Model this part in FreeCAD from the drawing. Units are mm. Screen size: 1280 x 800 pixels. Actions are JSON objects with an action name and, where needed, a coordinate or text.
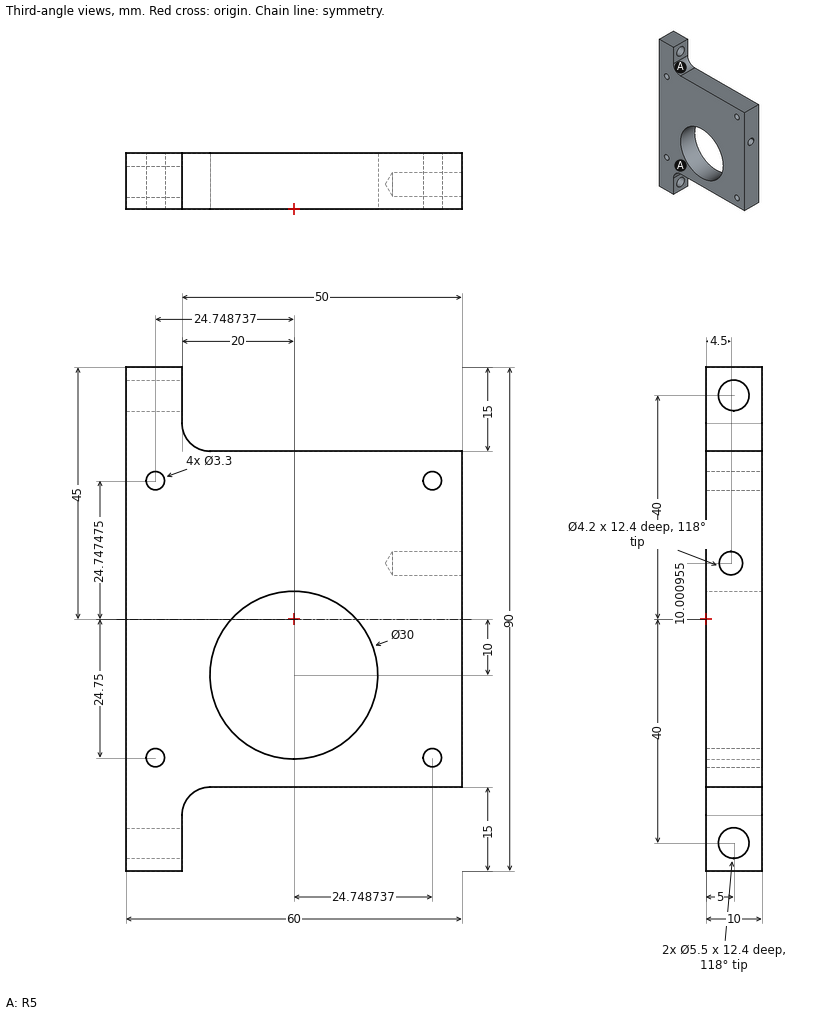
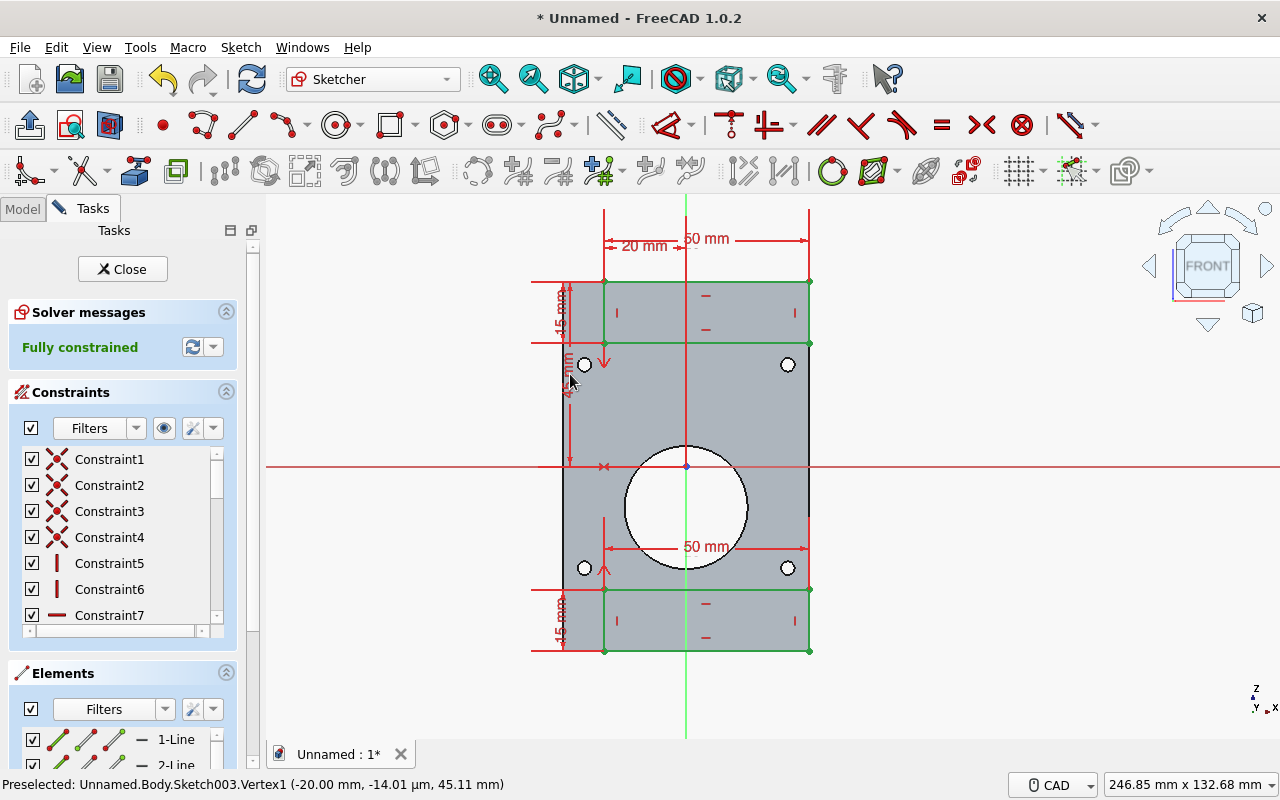
{"action": "left_click", "coordinate": [123, 269]}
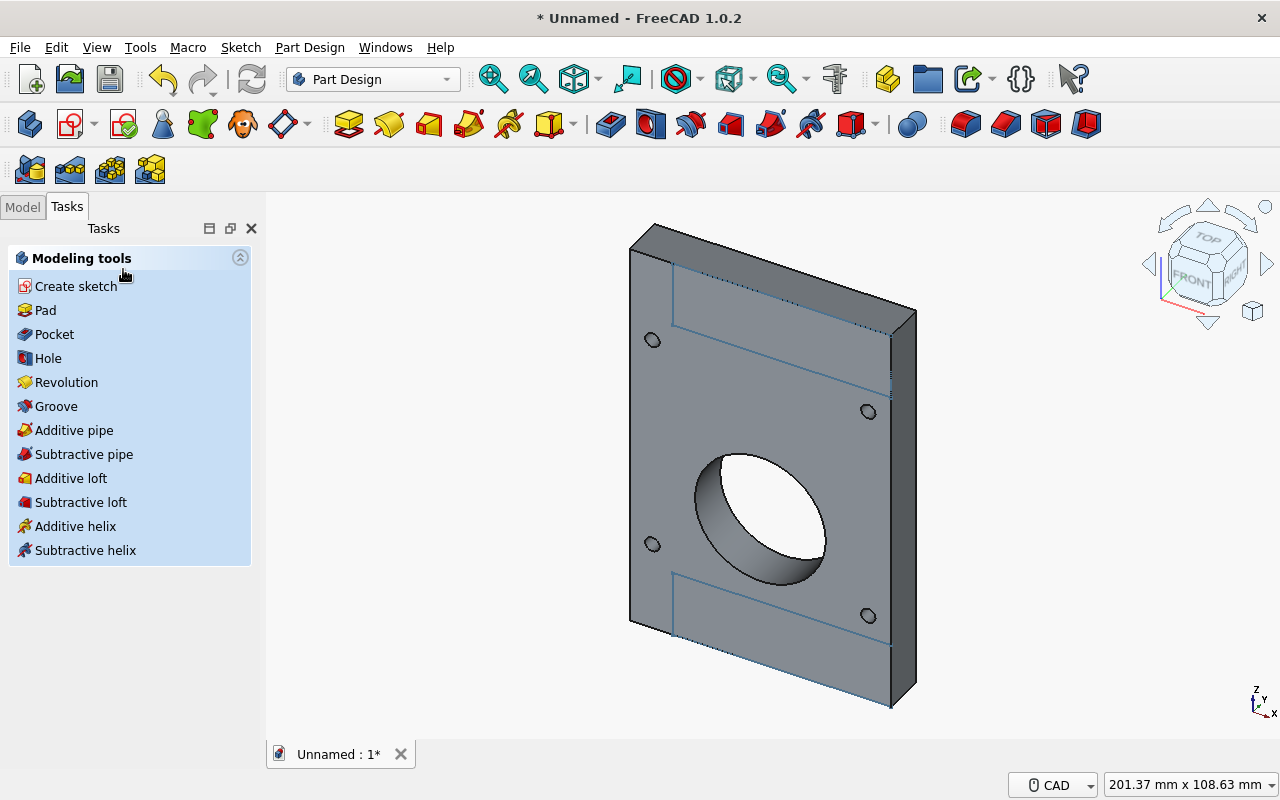
{"action": "left_click", "coordinate": [612, 124]}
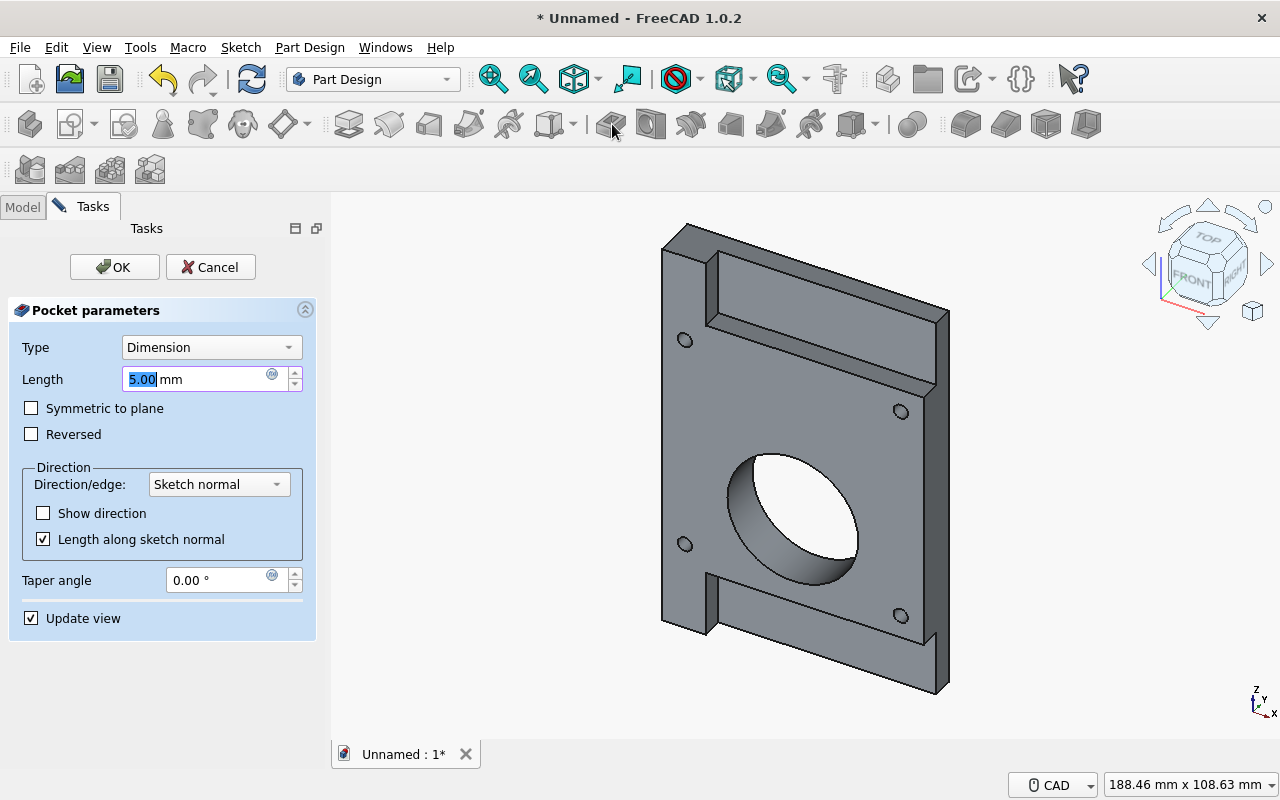
{"action": "left_click", "coordinate": [212, 348]}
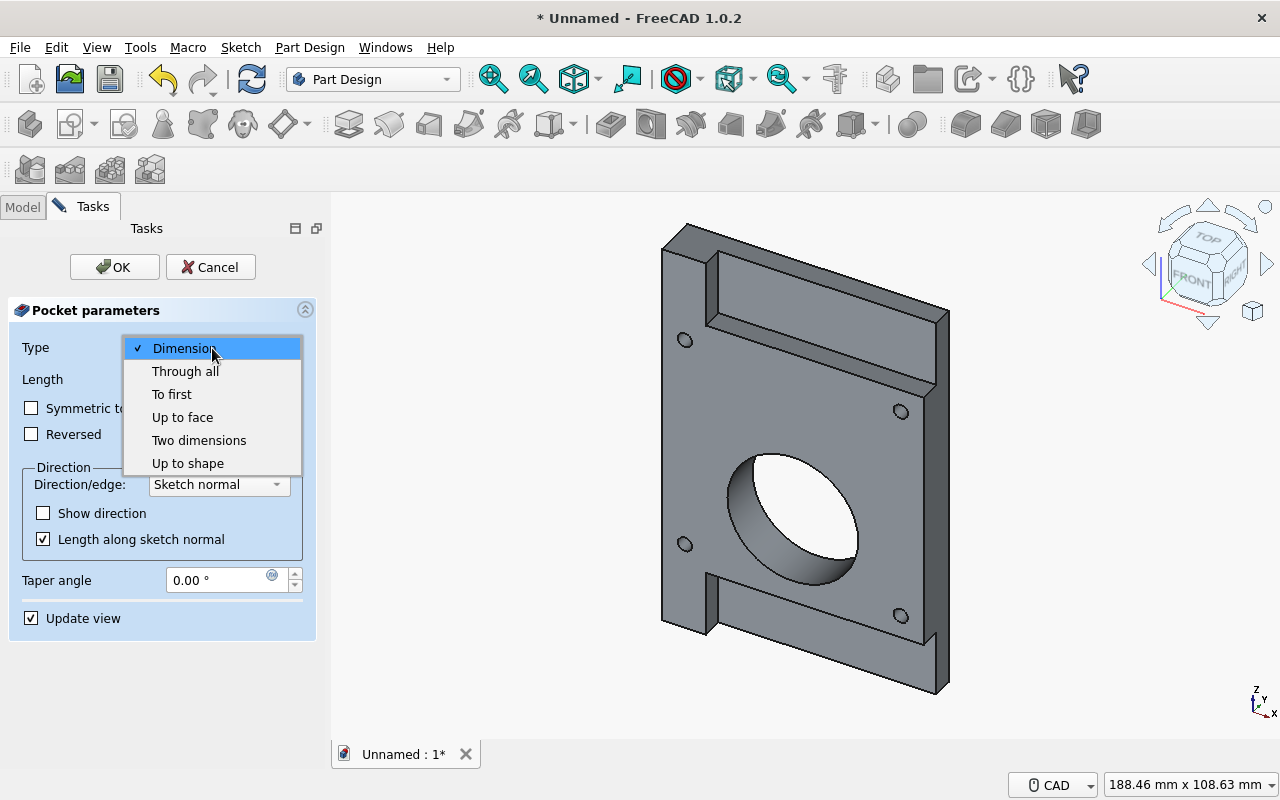
{"action": "left_click", "coordinate": [212, 372]}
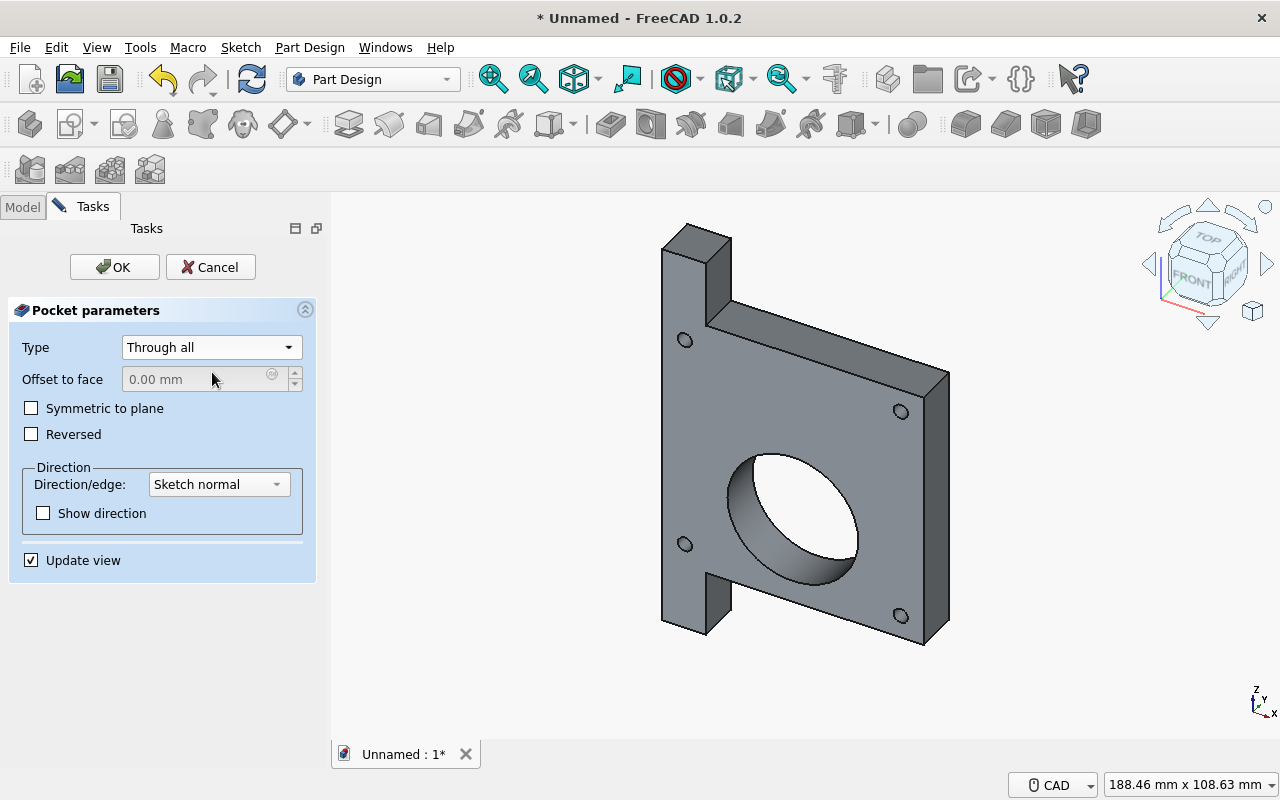
{"action": "left_click", "coordinate": [115, 267]}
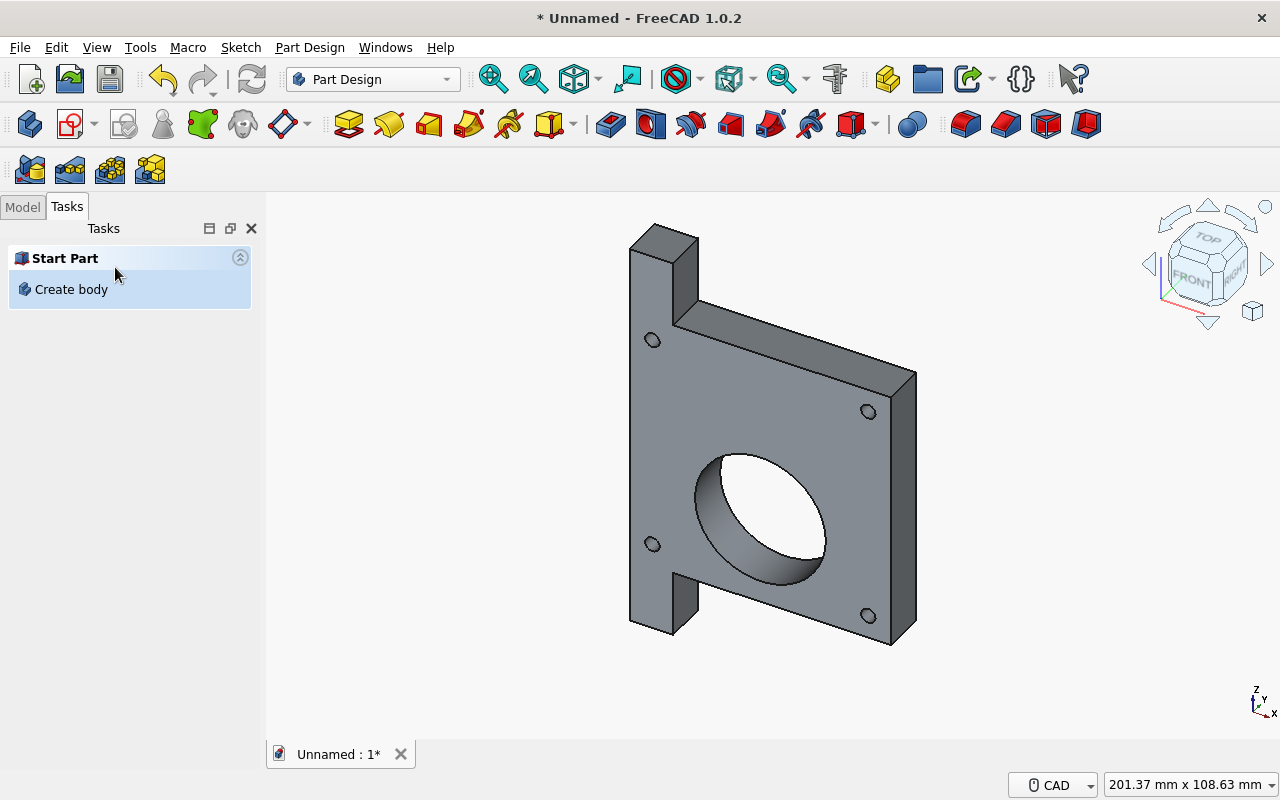
{"action": "key", "text": "6"}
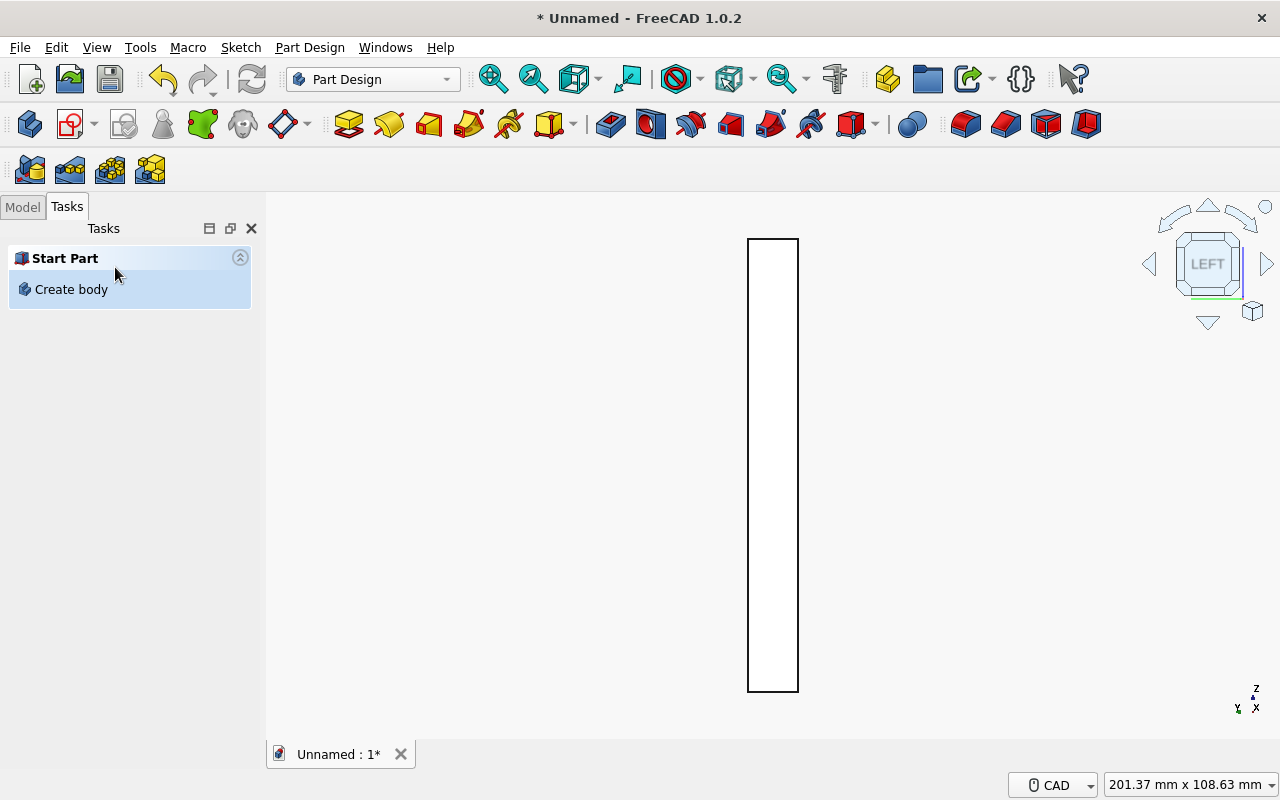
{"action": "left_click", "coordinate": [773, 270]}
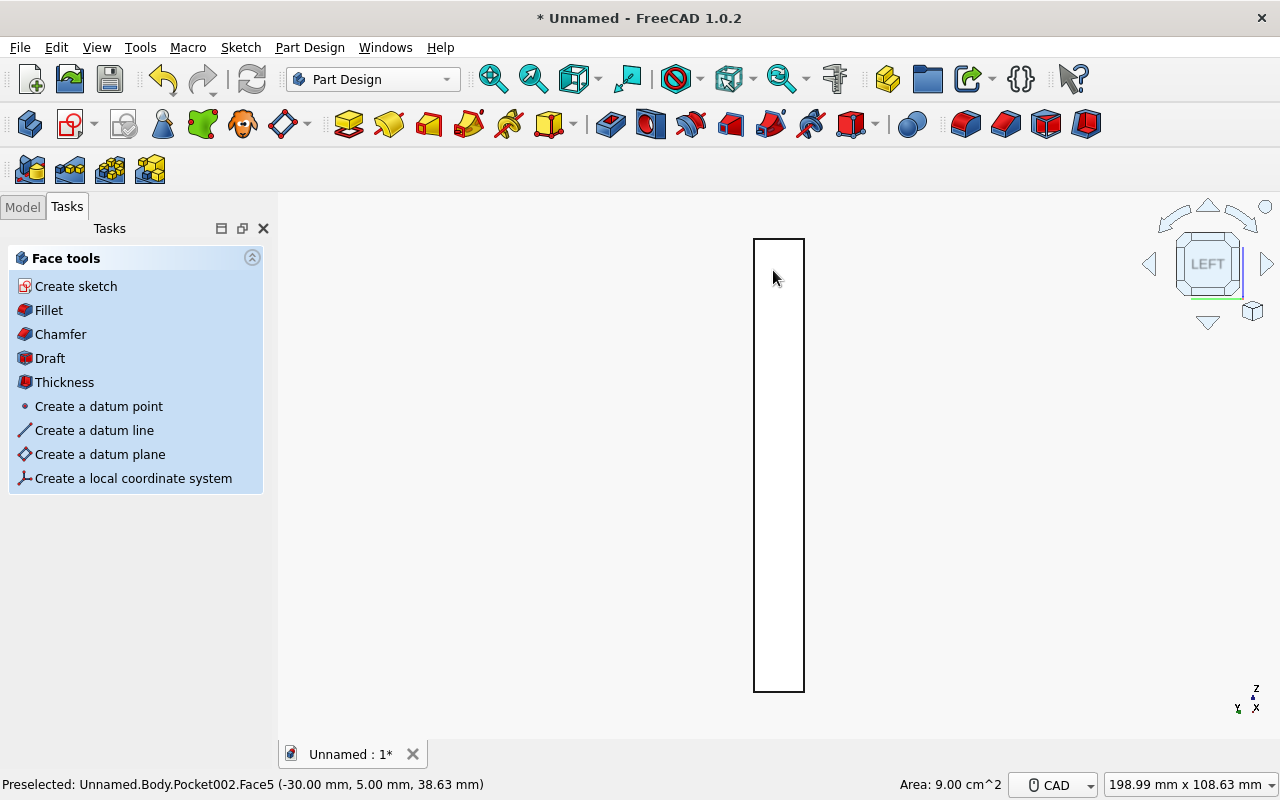
{"action": "left_click", "coordinate": [70, 124]}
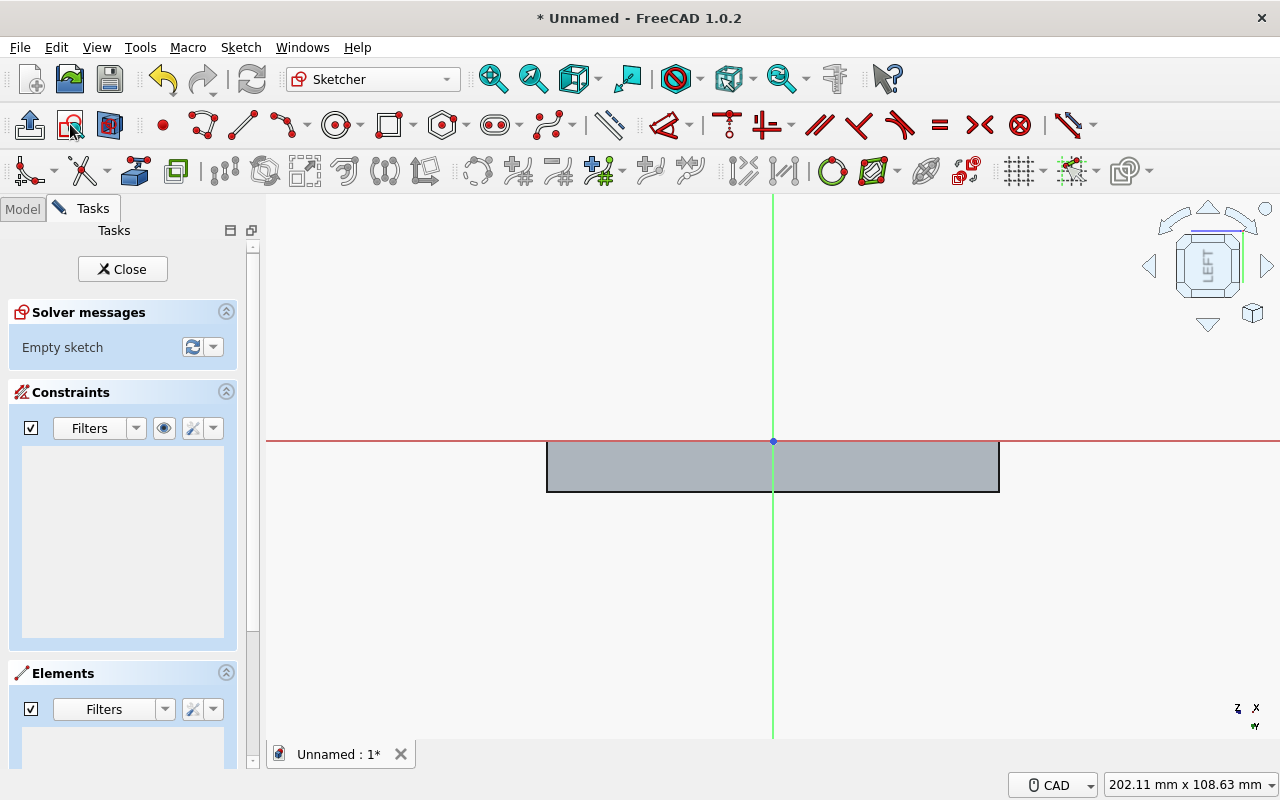
{"action": "scroll", "coordinate": [912, 449], "scroll_direction": "up", "scroll_amount": 2}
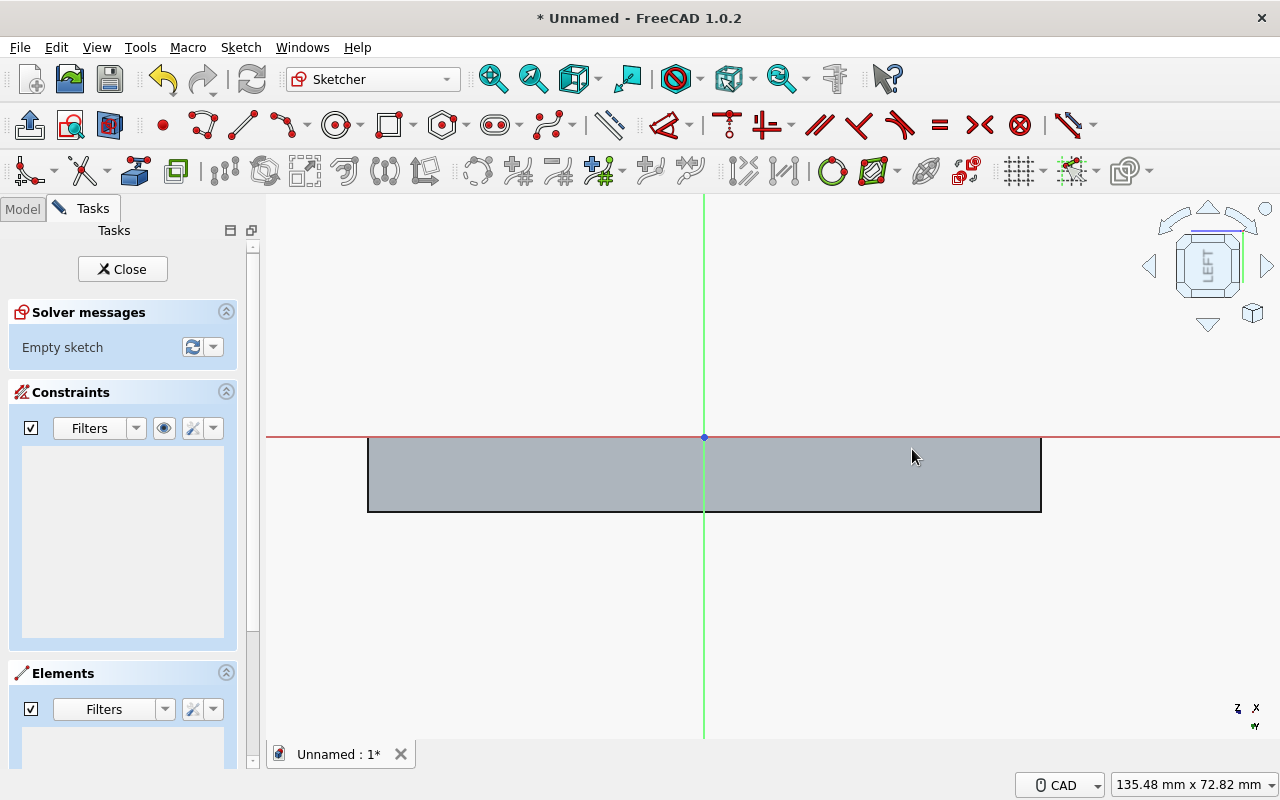
{"action": "key", "text": "g c"}